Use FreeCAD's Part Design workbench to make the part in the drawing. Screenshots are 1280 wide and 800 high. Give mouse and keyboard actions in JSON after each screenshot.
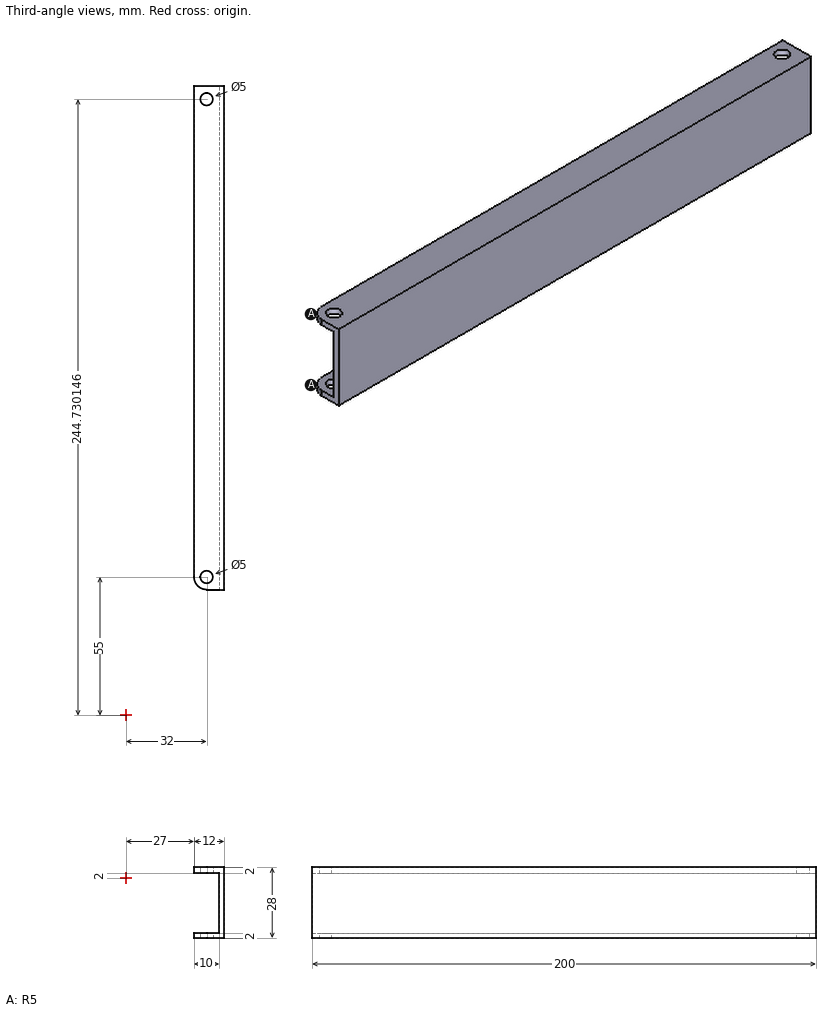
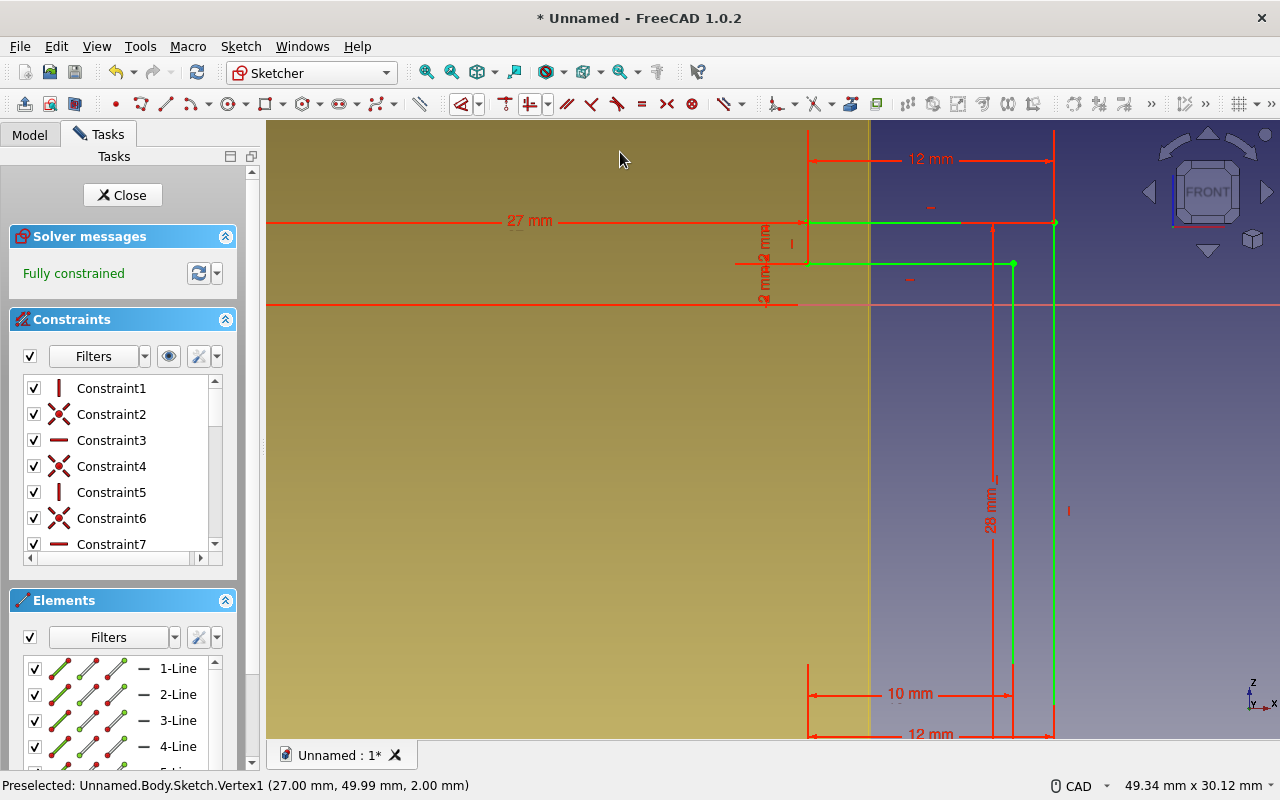
{"action": "left_click", "coordinate": [123, 195]}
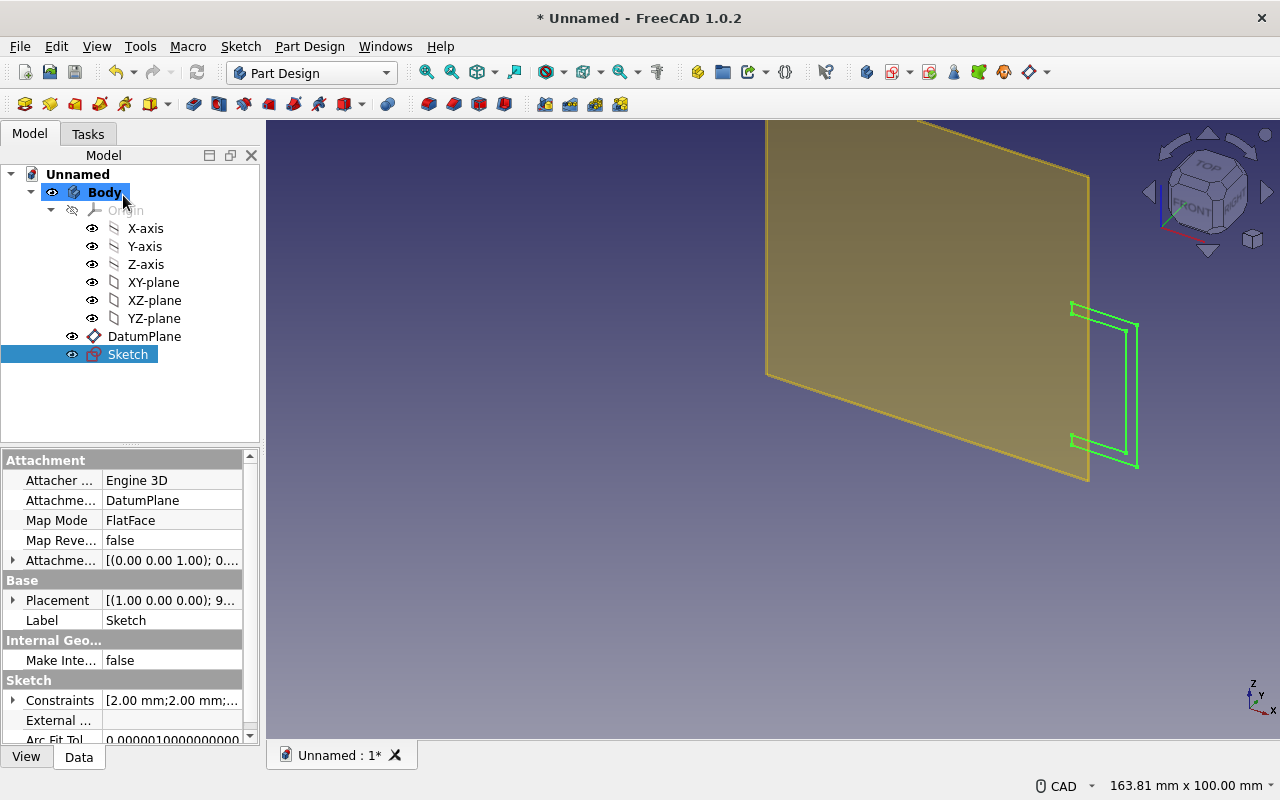
{"action": "left_click", "coordinate": [25, 104]}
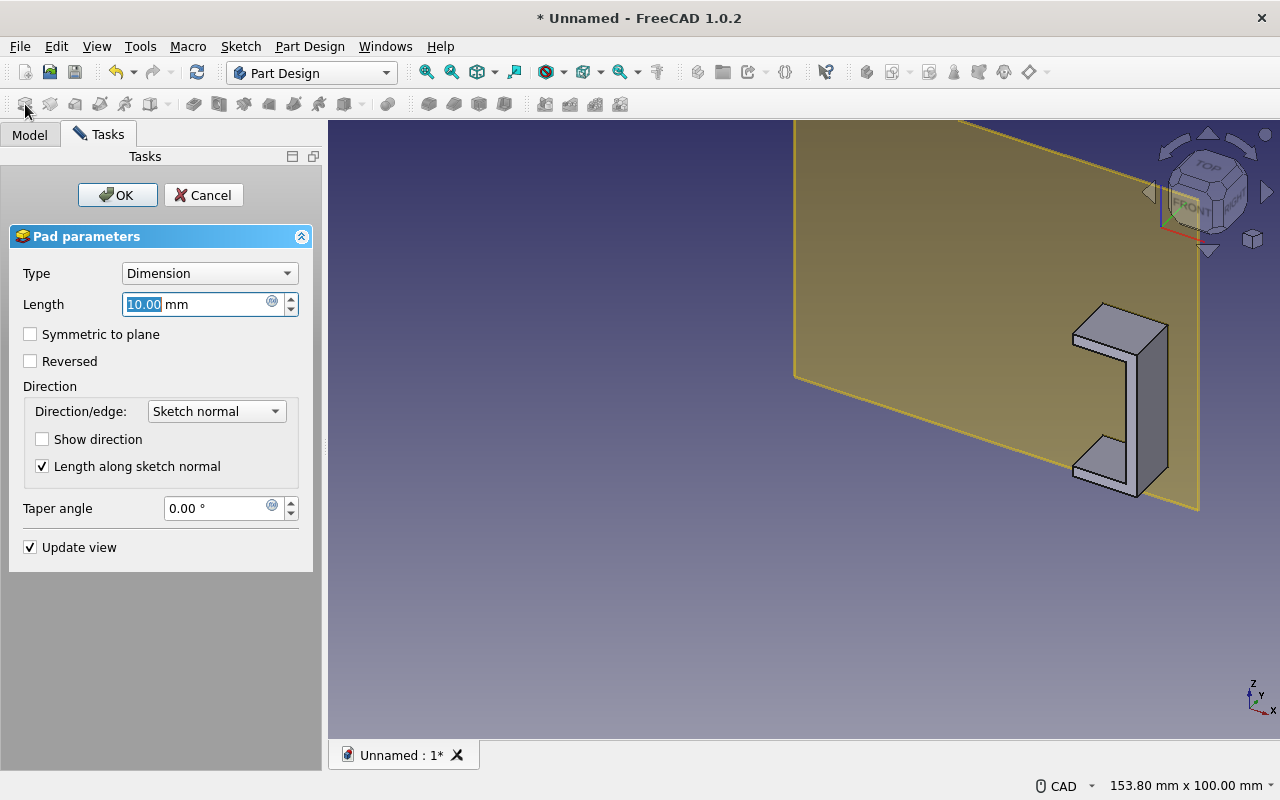
{"action": "type", "text": "200"}
{"action": "key", "text": "Tab"}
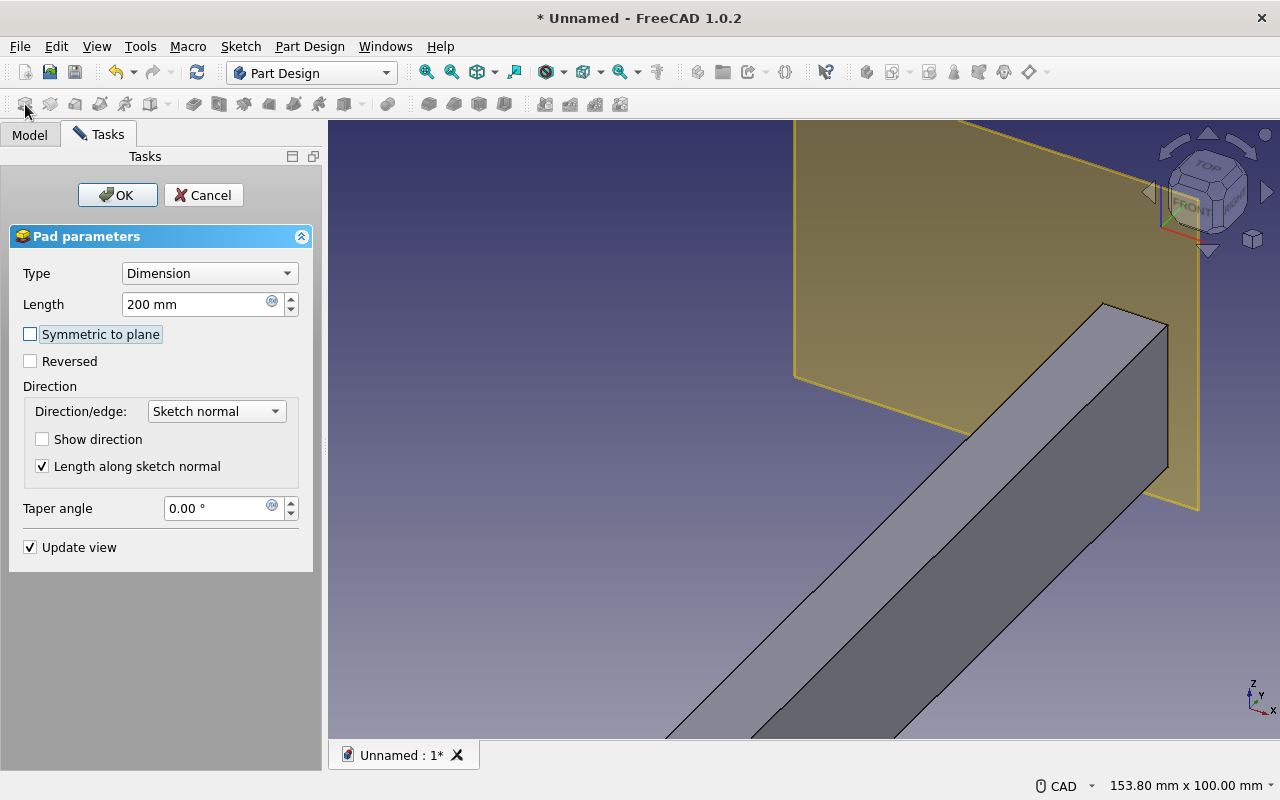
{"action": "left_click", "coordinate": [31, 361]}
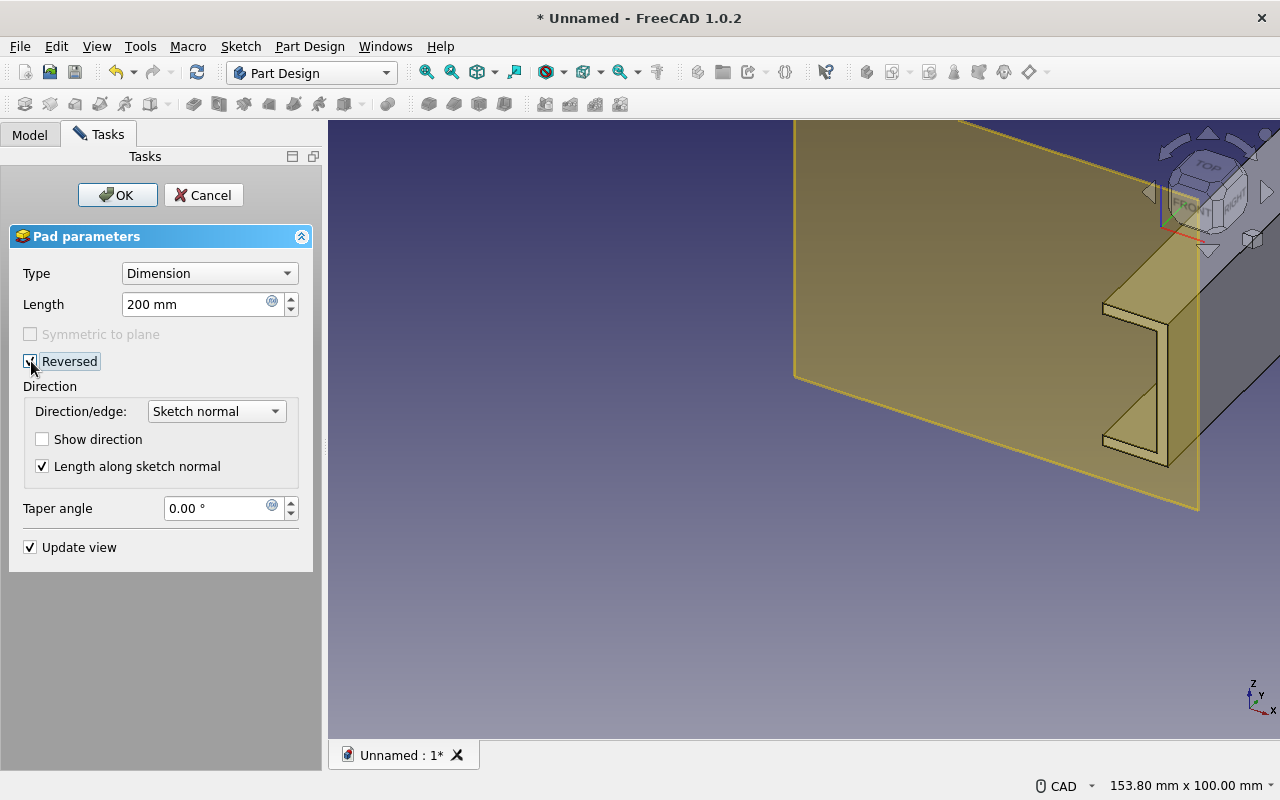
{"action": "left_click", "coordinate": [118, 195]}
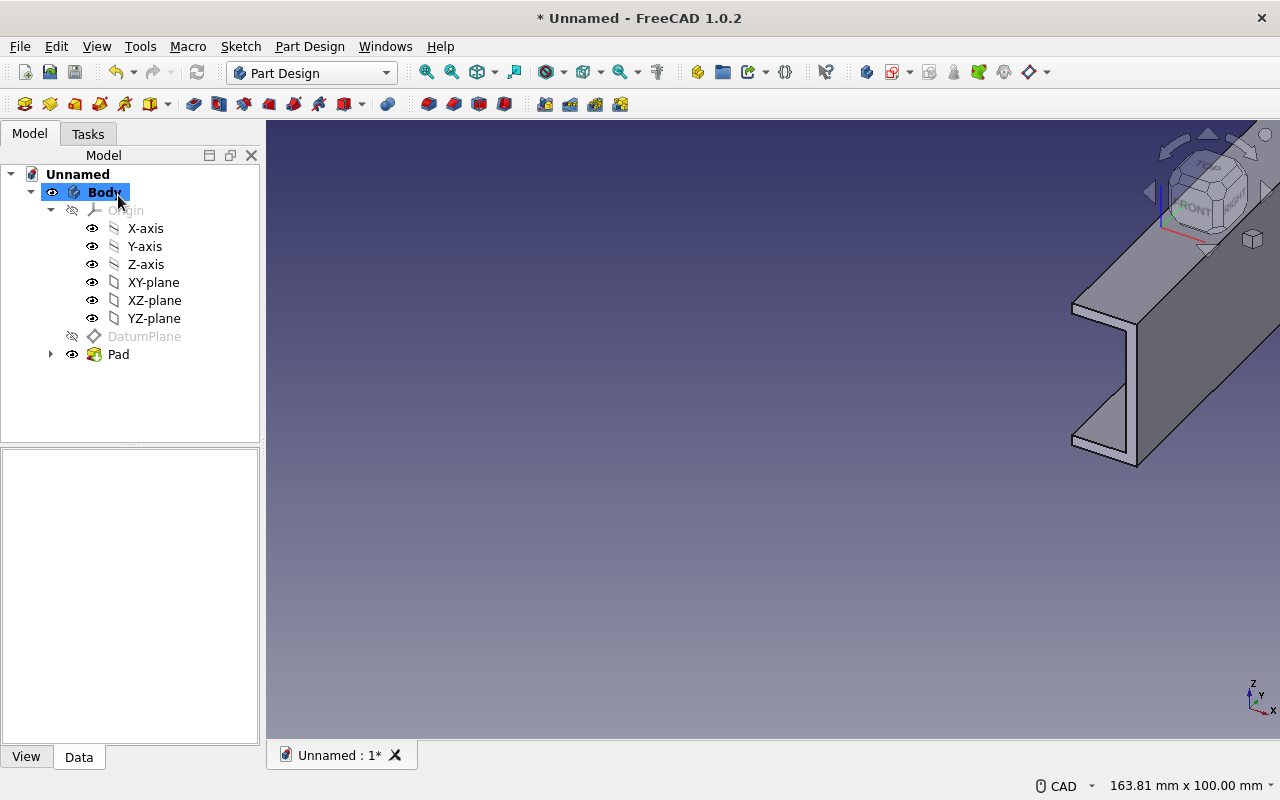
{"action": "left_click", "coordinate": [427, 72]}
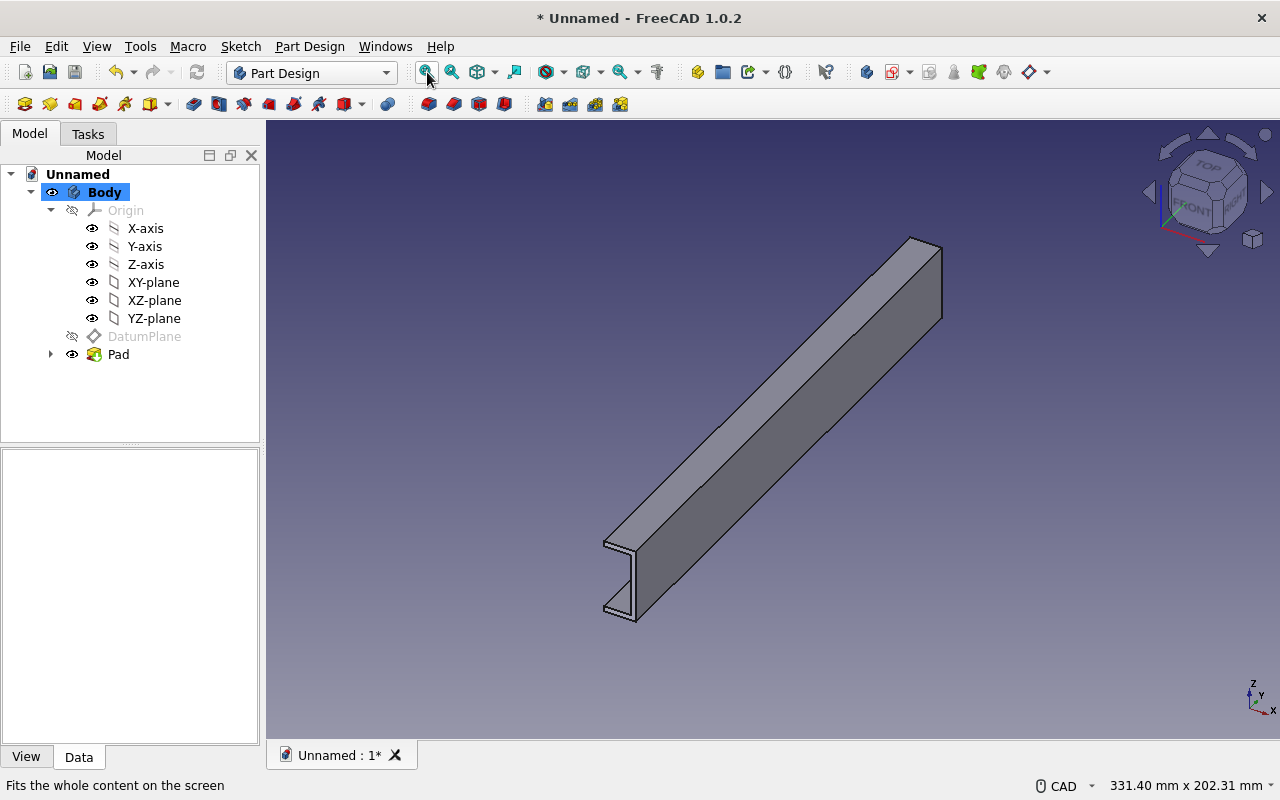
{"action": "scroll", "coordinate": [604, 543], "scroll_direction": "up", "scroll_amount": 10}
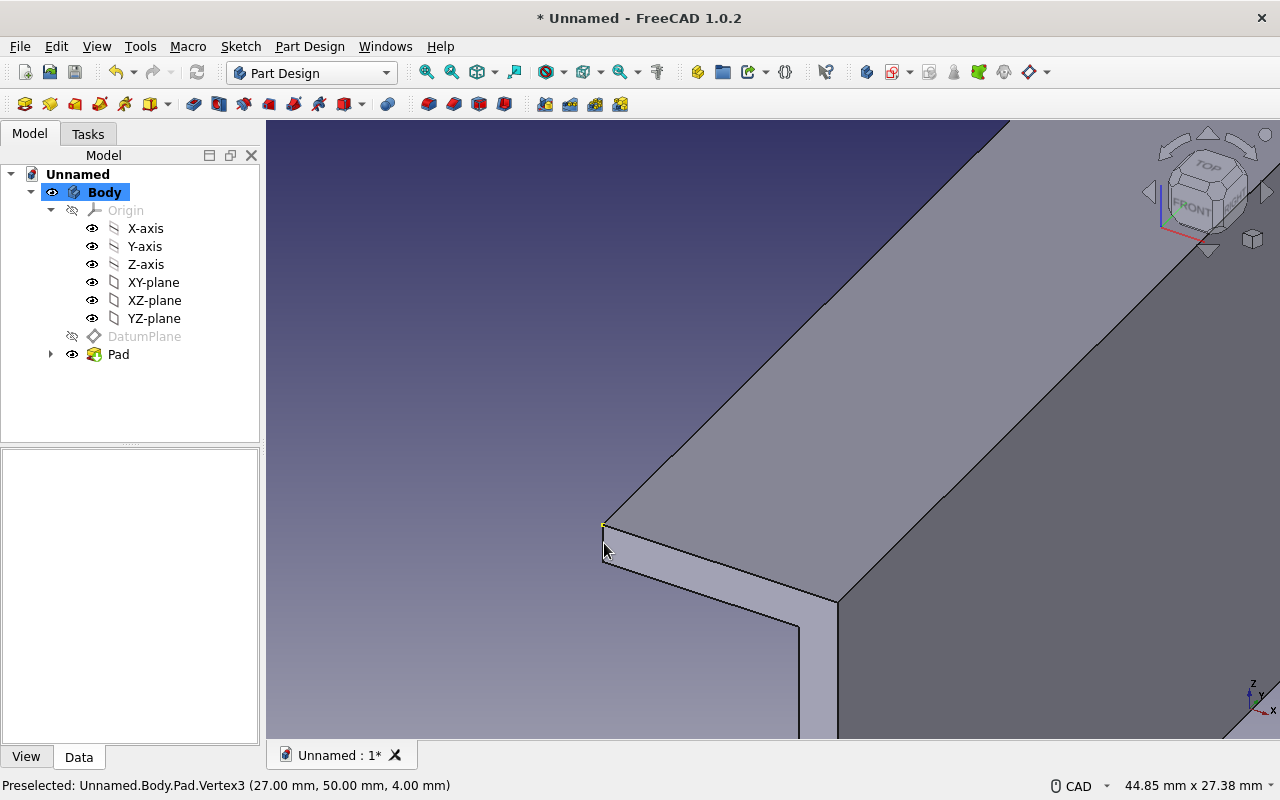
{"action": "left_click", "coordinate": [427, 72]}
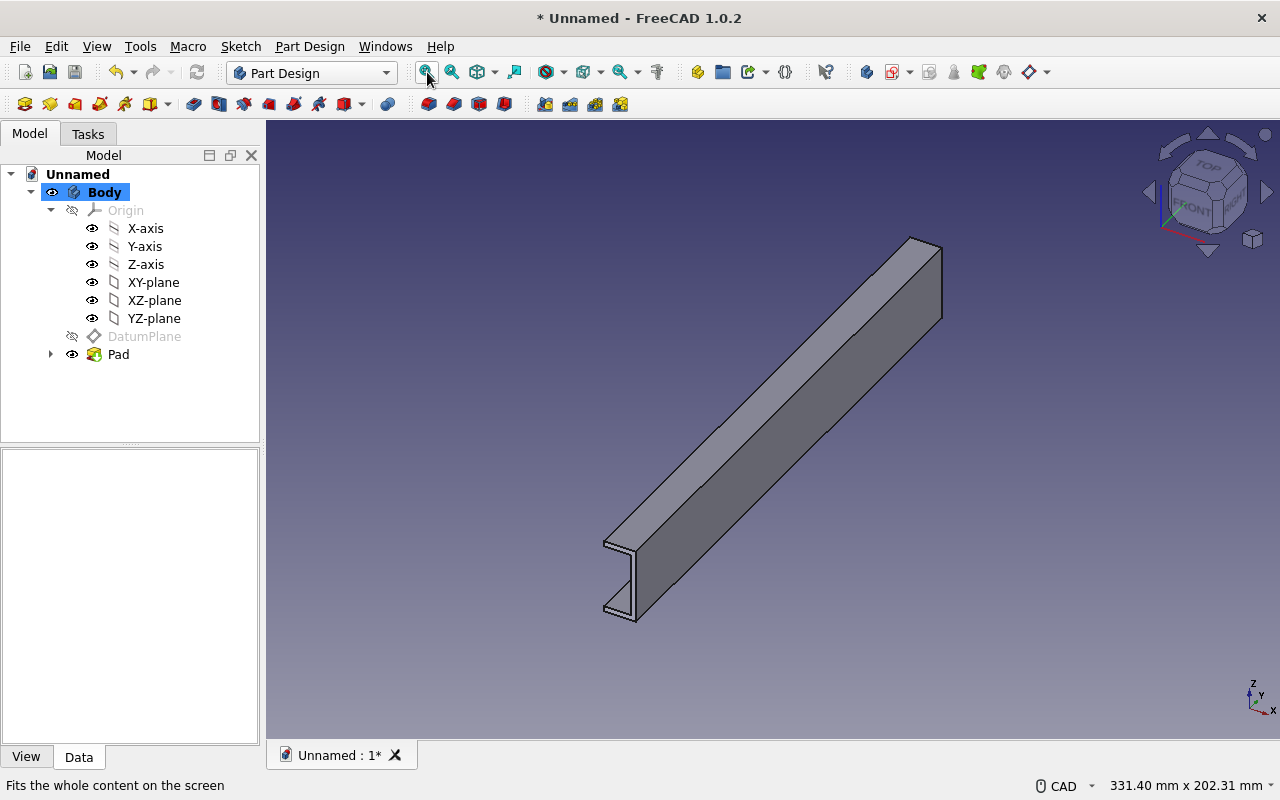
{"action": "key", "text": "0"}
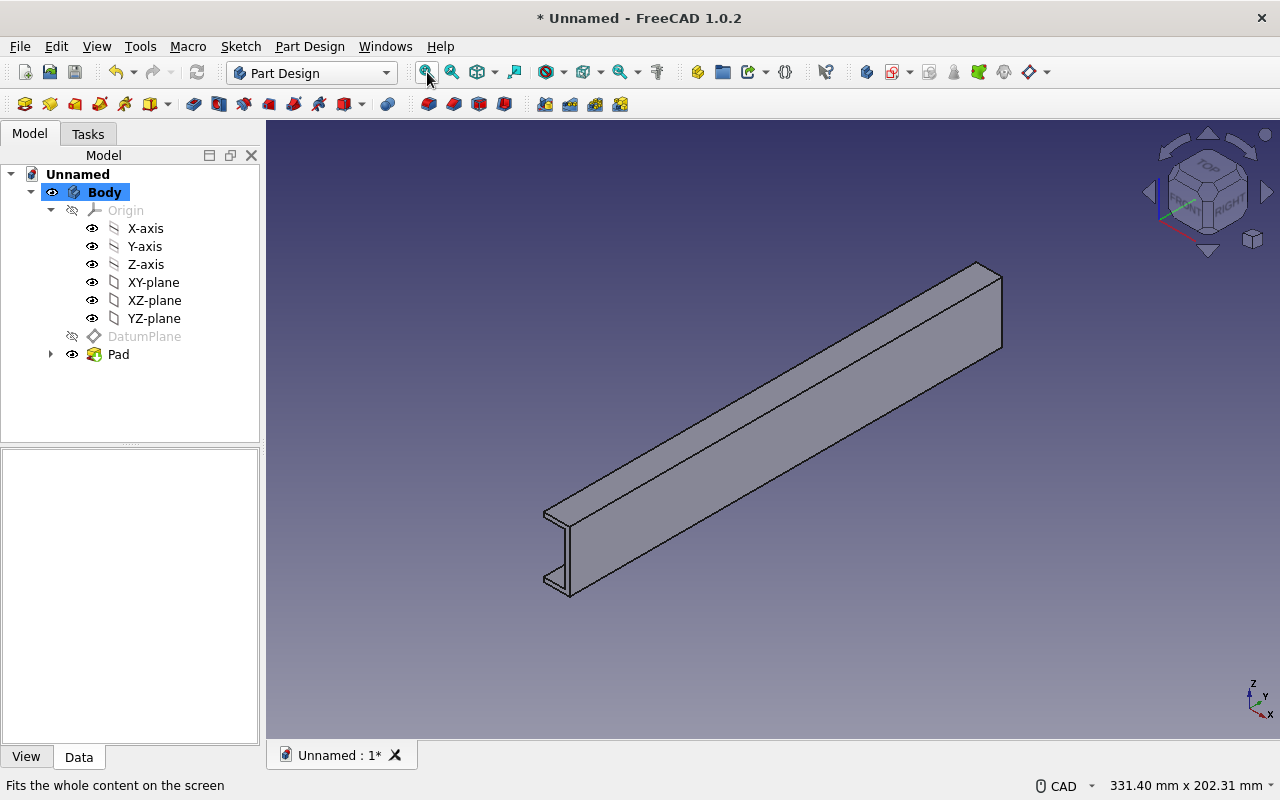
{"action": "scroll", "coordinate": [544, 513], "scroll_direction": "up", "scroll_amount": 10}